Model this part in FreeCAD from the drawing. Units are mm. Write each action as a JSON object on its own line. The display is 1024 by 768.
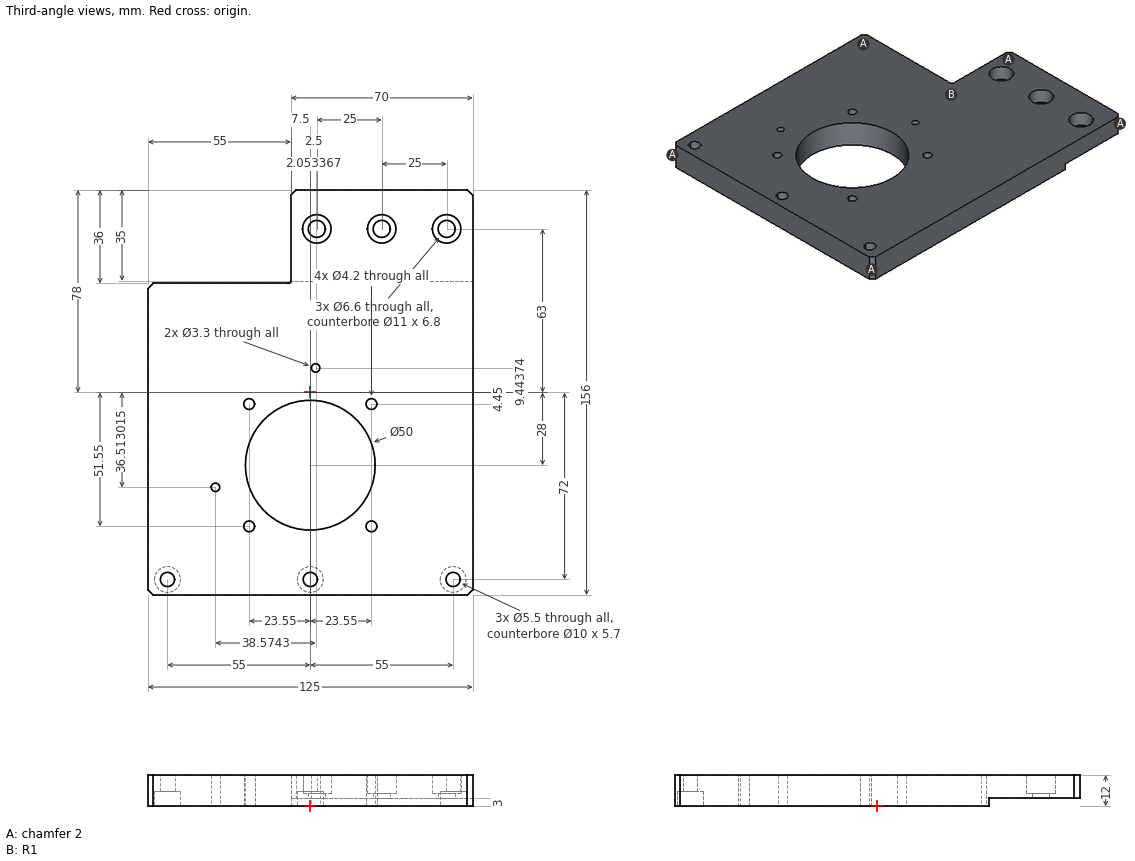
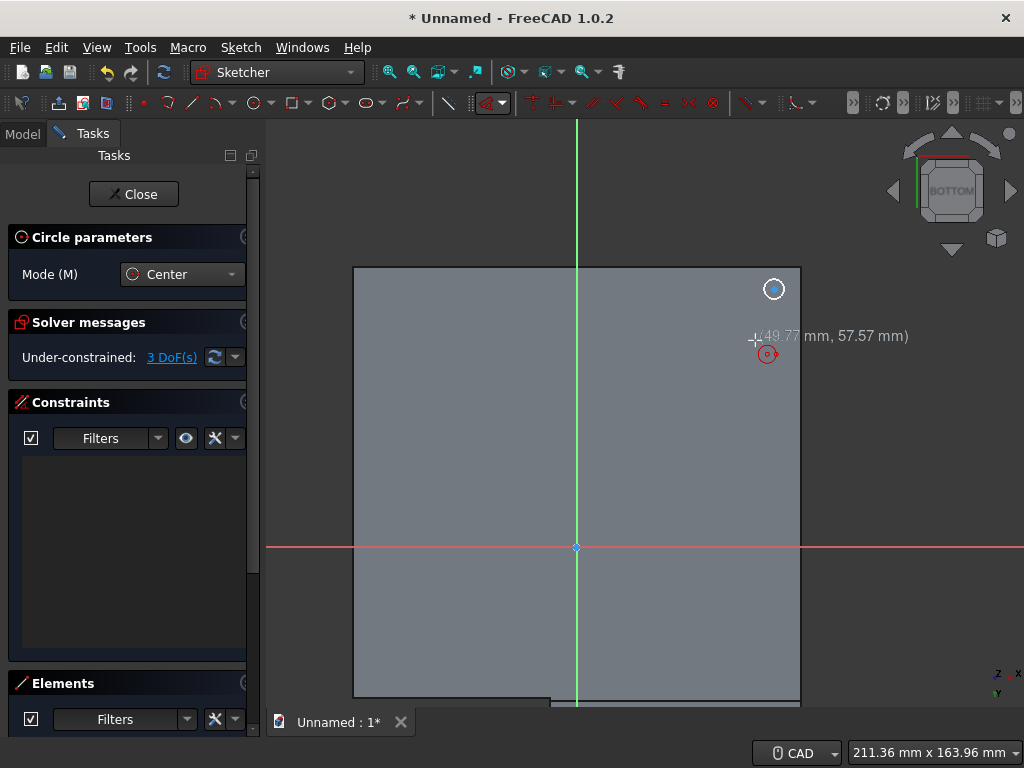
{"action": "scroll", "coordinate": [577, 289], "scroll_direction": "up", "scroll_amount": 5}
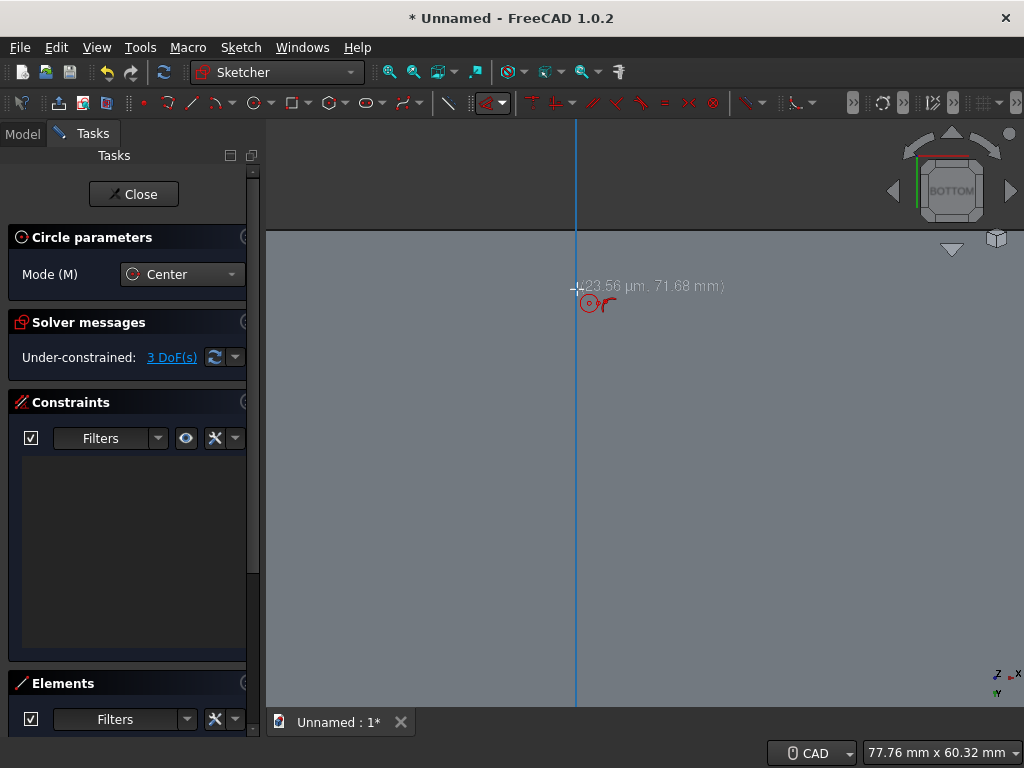
{"action": "left_click", "coordinate": [576, 288]}
{"action": "left_click", "coordinate": [595, 269]}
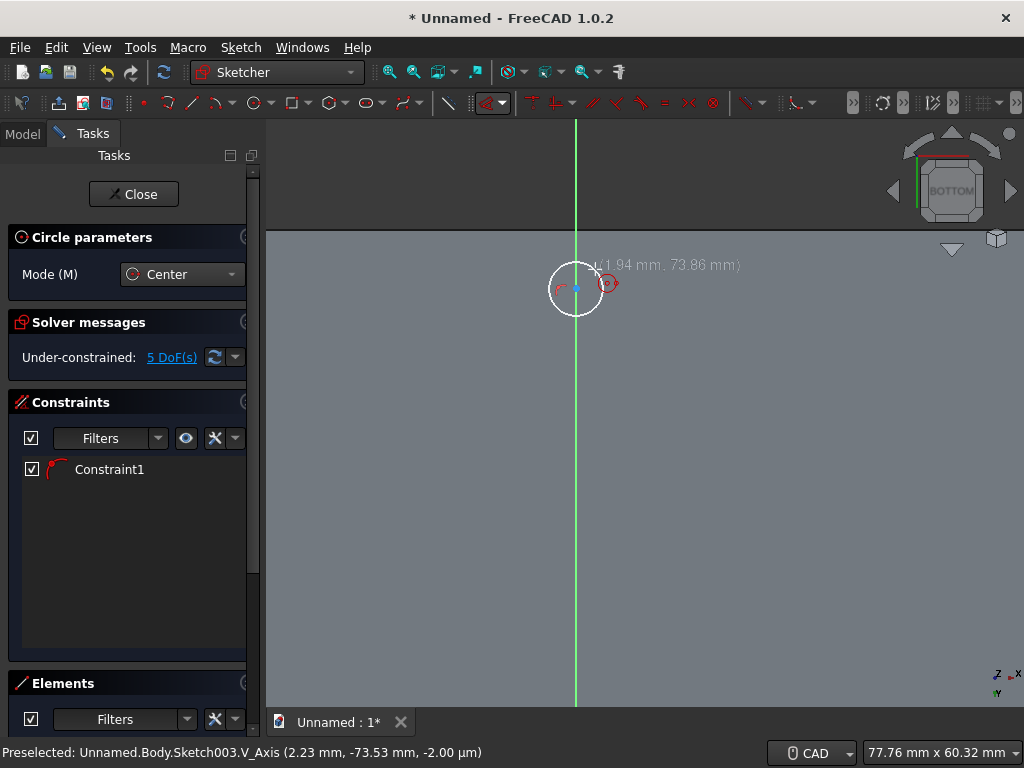
{"action": "scroll", "coordinate": [577, 289], "scroll_direction": "down", "scroll_amount": 5}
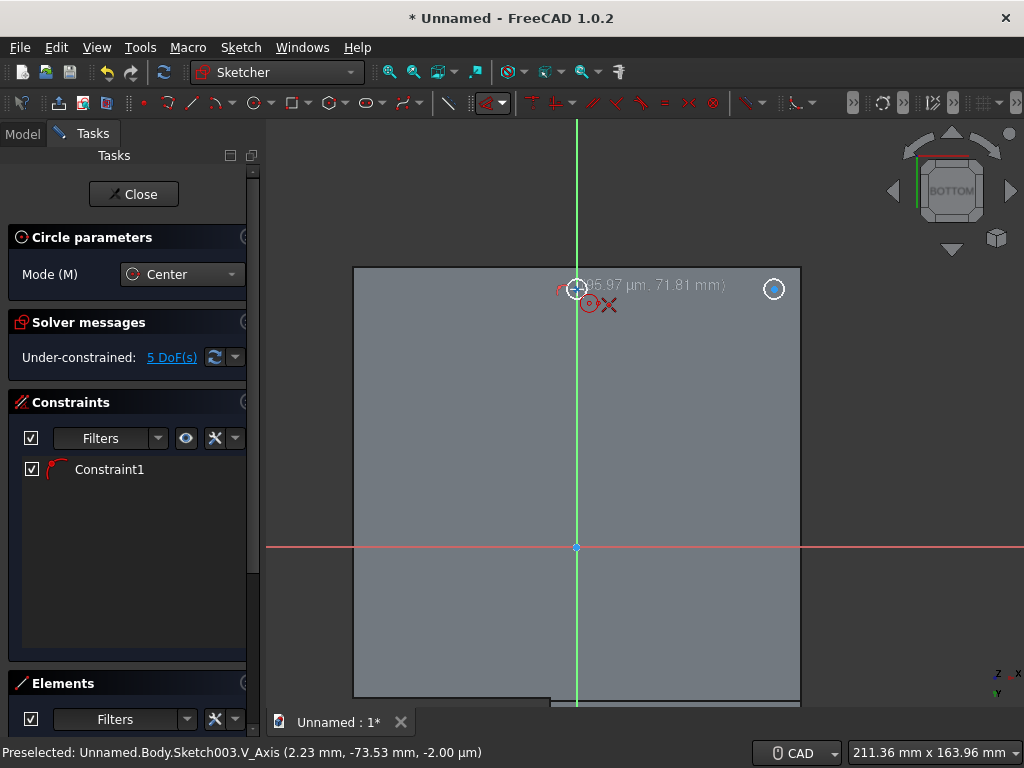
{"action": "scroll", "coordinate": [380, 289], "scroll_direction": "up", "scroll_amount": 5}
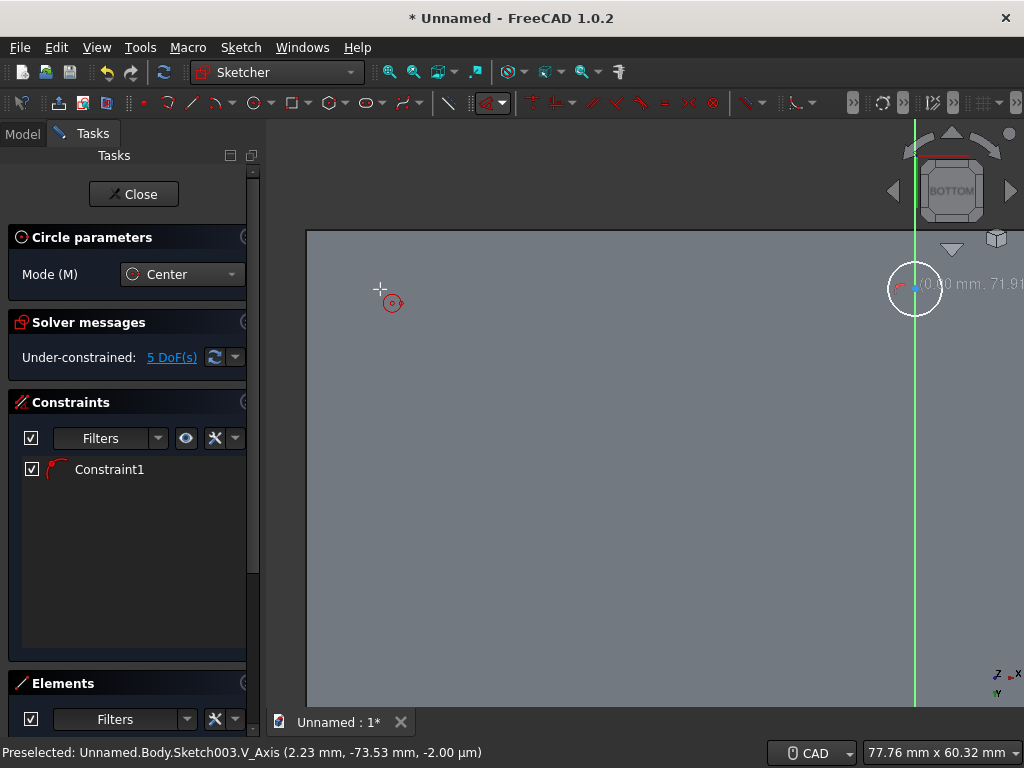
{"action": "left_click", "coordinate": [379, 288]}
{"action": "left_click", "coordinate": [398, 269]}
{"action": "key", "text": "Escape"}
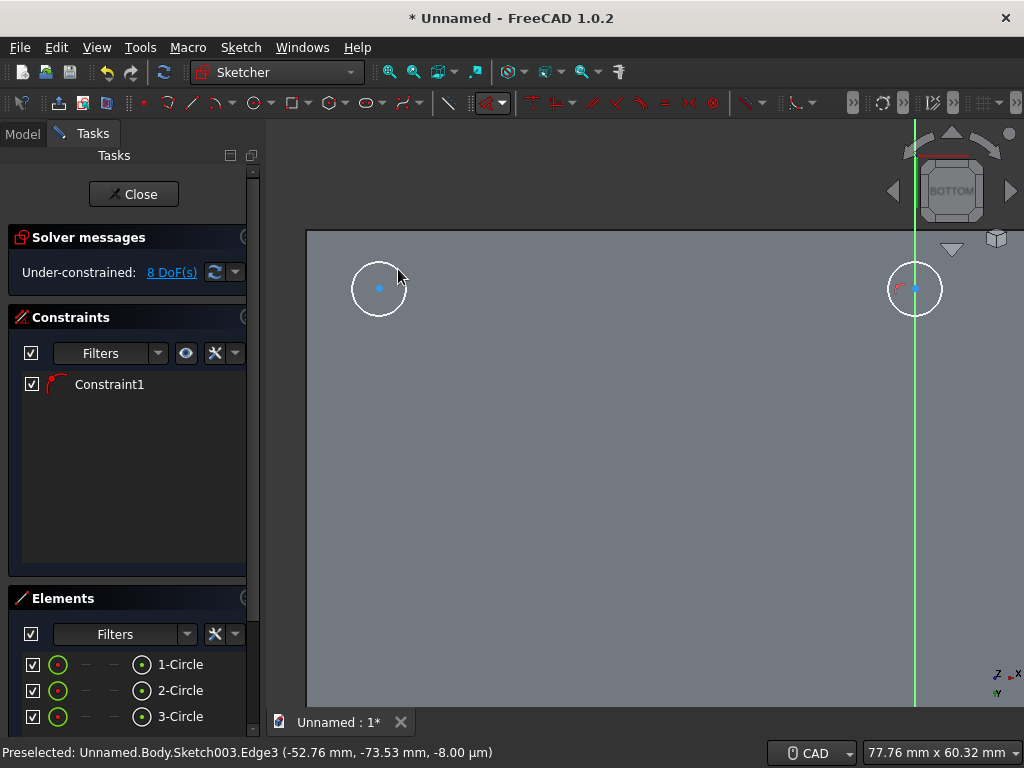
{"action": "scroll", "coordinate": [379, 289], "scroll_direction": "down", "scroll_amount": 5}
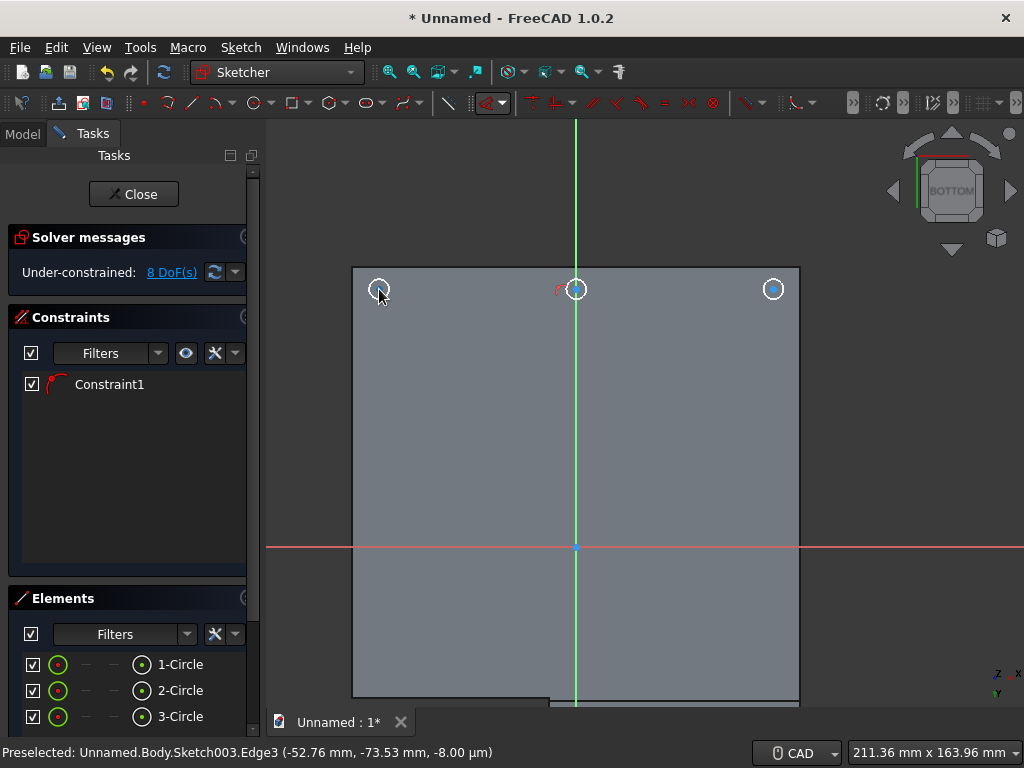
{"action": "scroll", "coordinate": [781, 282], "scroll_direction": "up", "scroll_amount": 2}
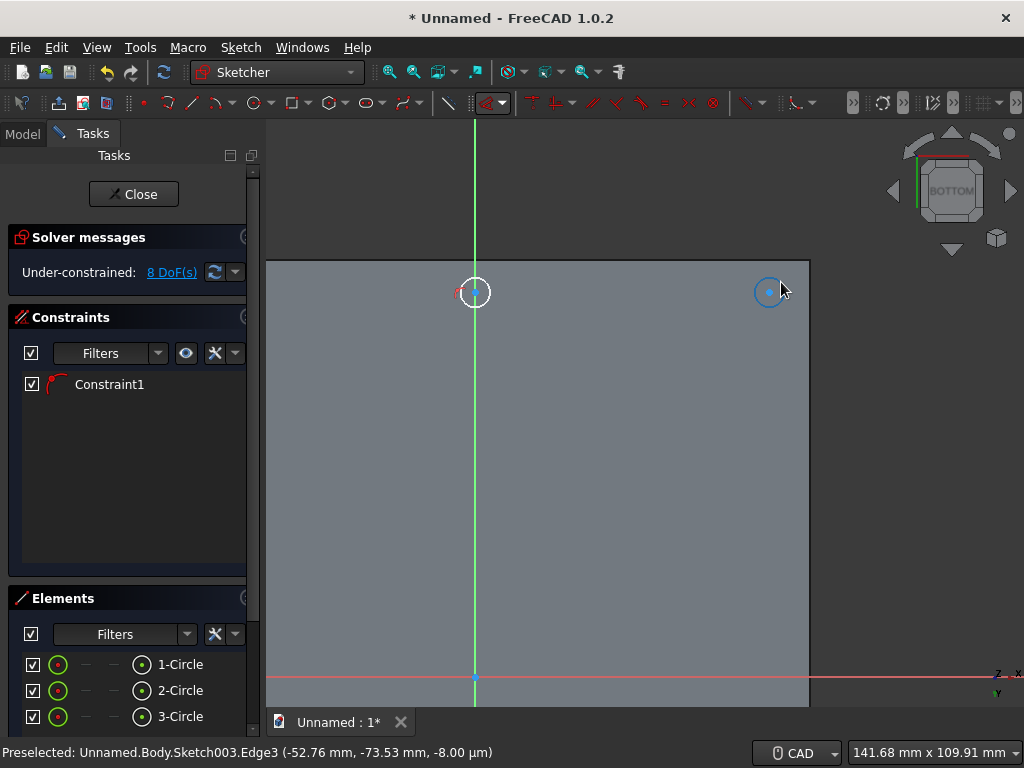
{"action": "left_click", "coordinate": [780, 282]}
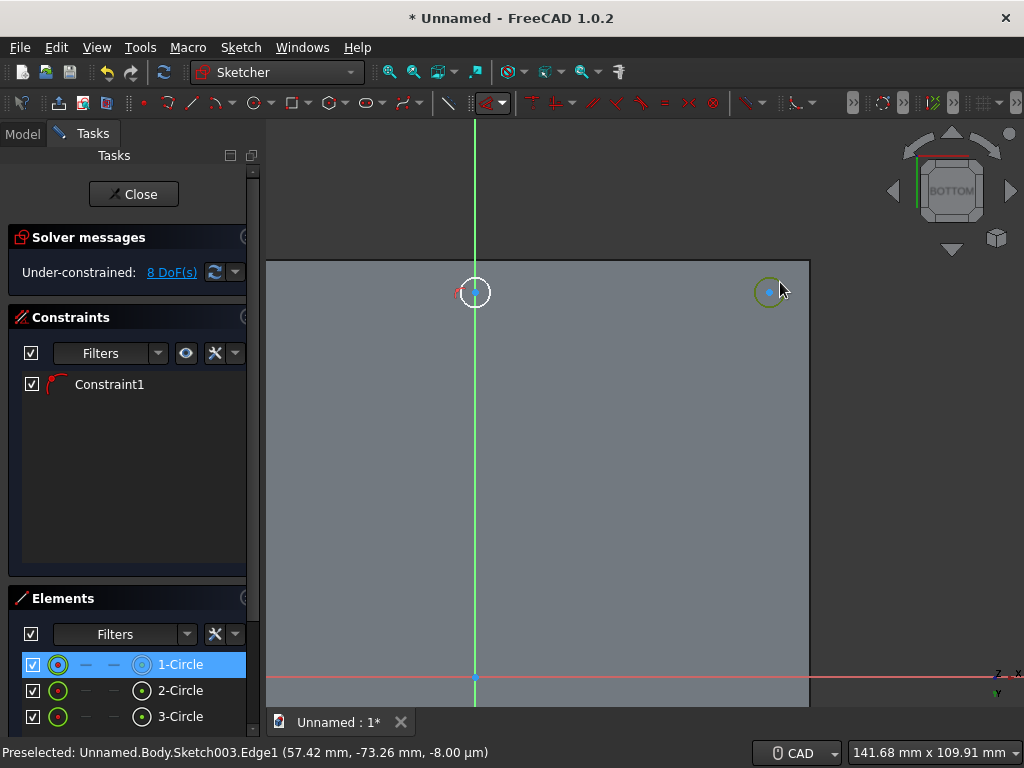
{"action": "scroll", "coordinate": [486, 282], "scroll_direction": "up", "scroll_amount": 2}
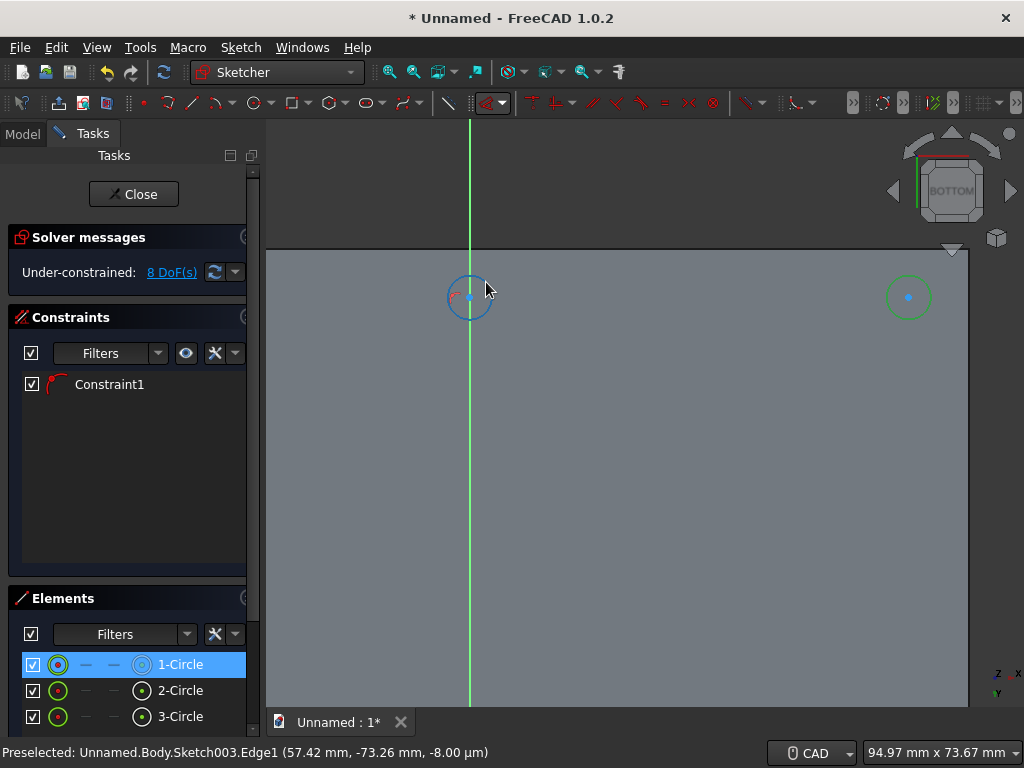
{"action": "left_click", "coordinate": [485, 282]}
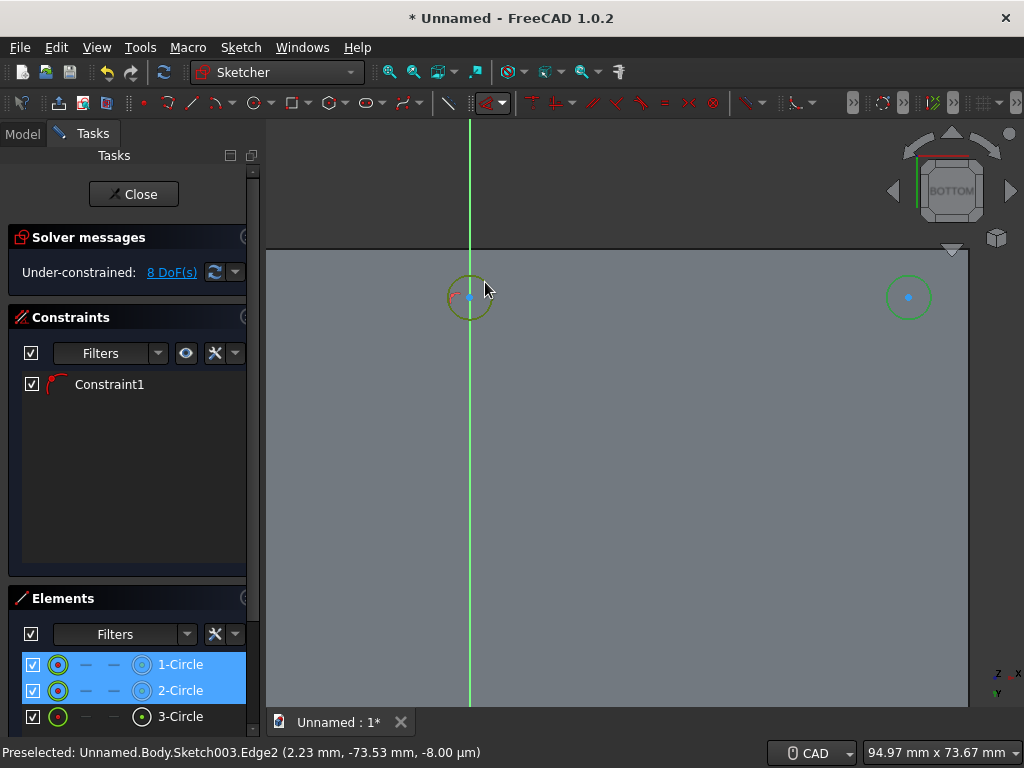
{"action": "scroll", "coordinate": [664, 282], "scroll_direction": "down", "scroll_amount": 4}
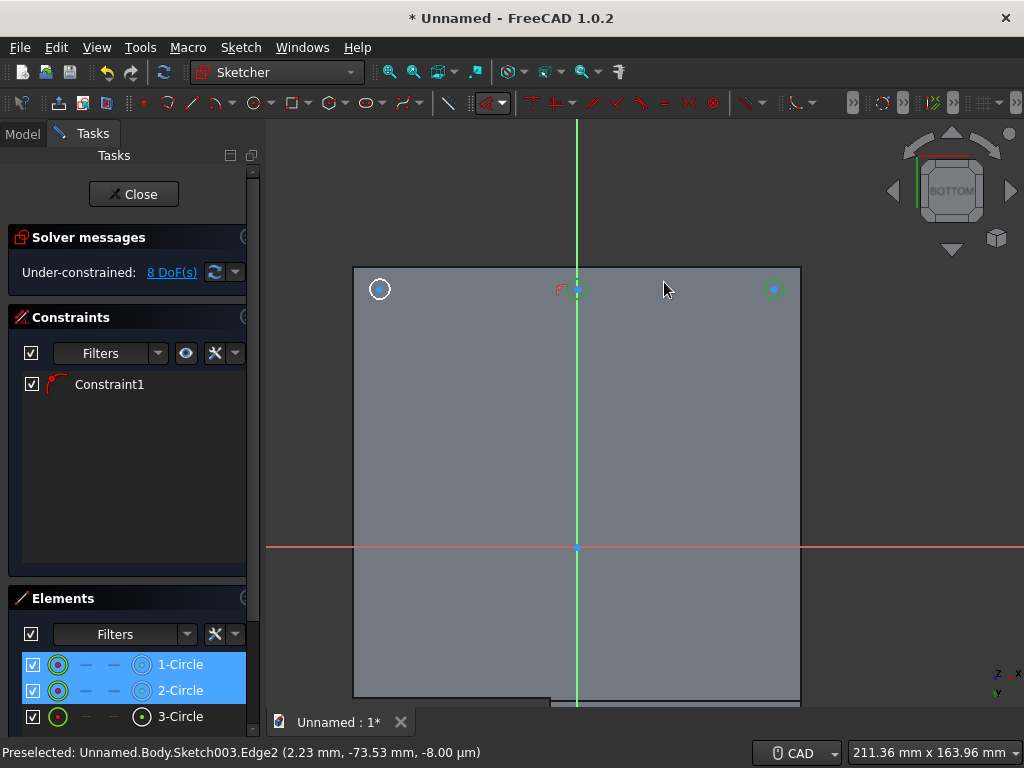
{"action": "scroll", "coordinate": [387, 282], "scroll_direction": "up", "scroll_amount": 2}